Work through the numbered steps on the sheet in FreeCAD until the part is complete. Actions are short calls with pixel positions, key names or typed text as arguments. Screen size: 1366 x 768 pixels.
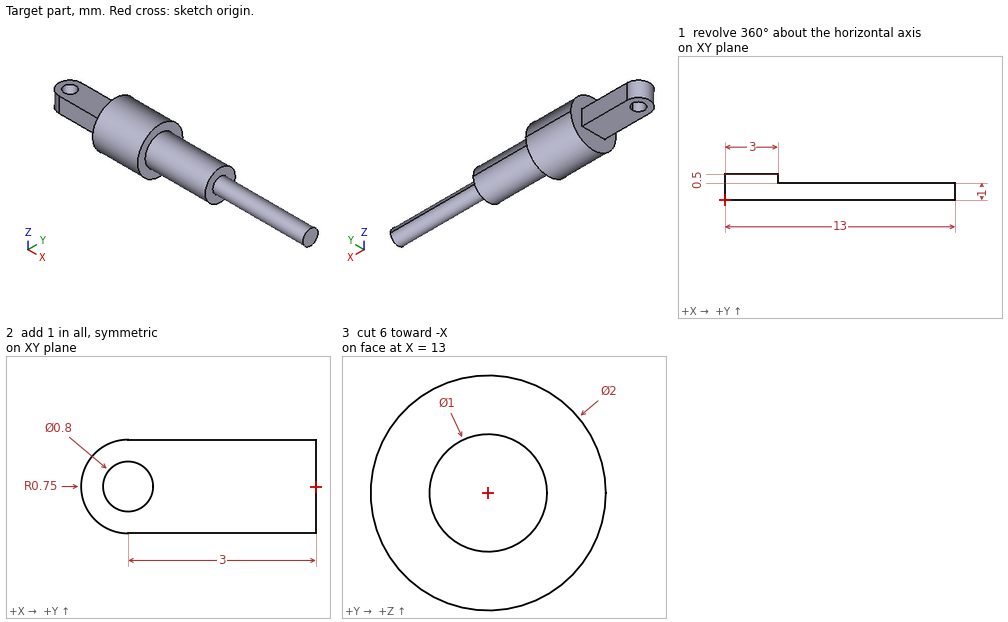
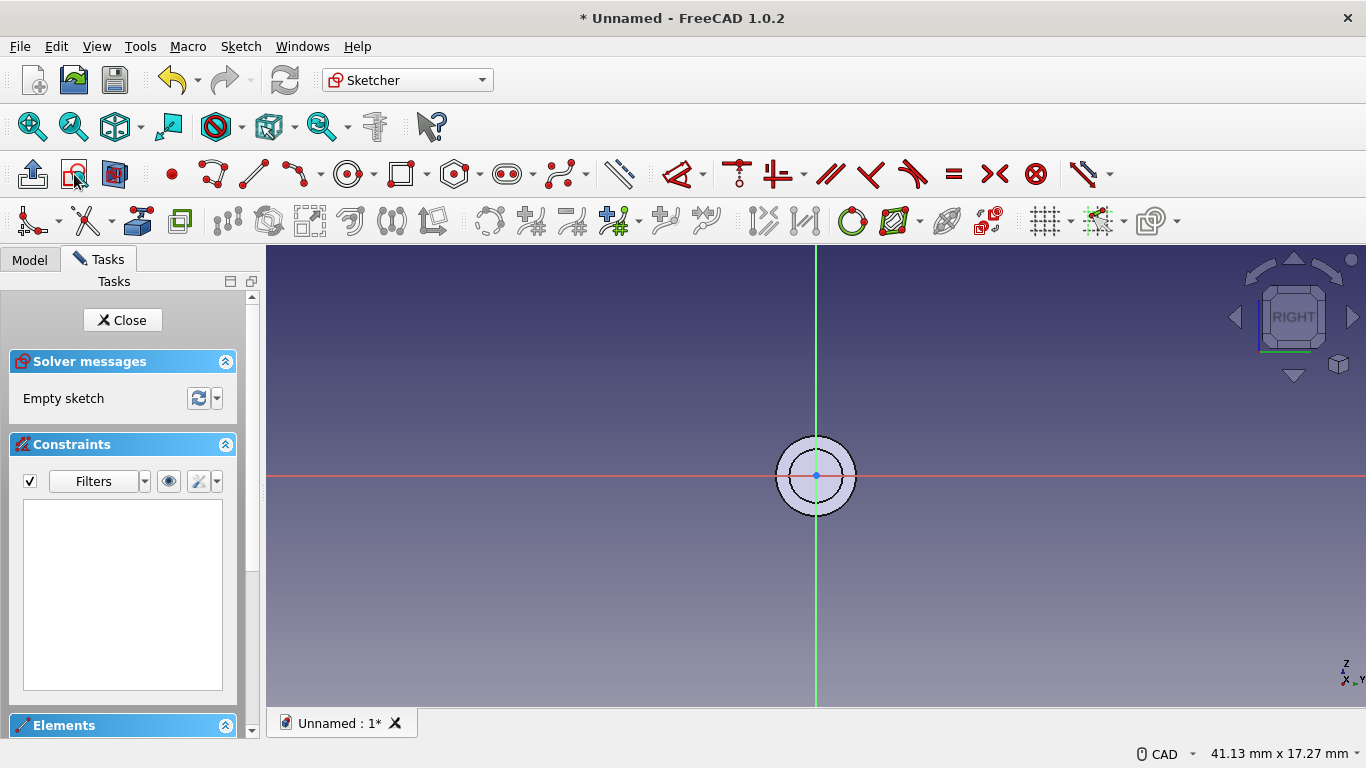
scroll(833, 476, up, 8)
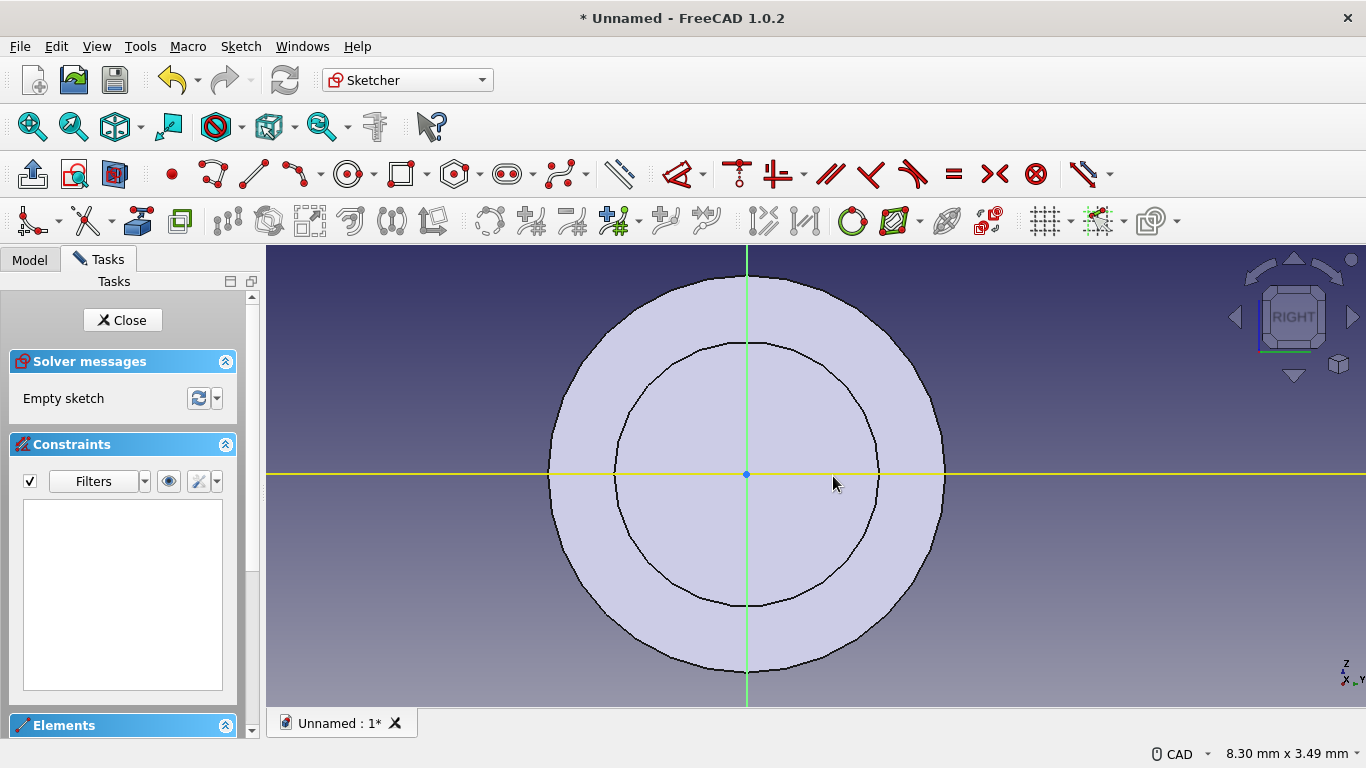
key(g)
key(c)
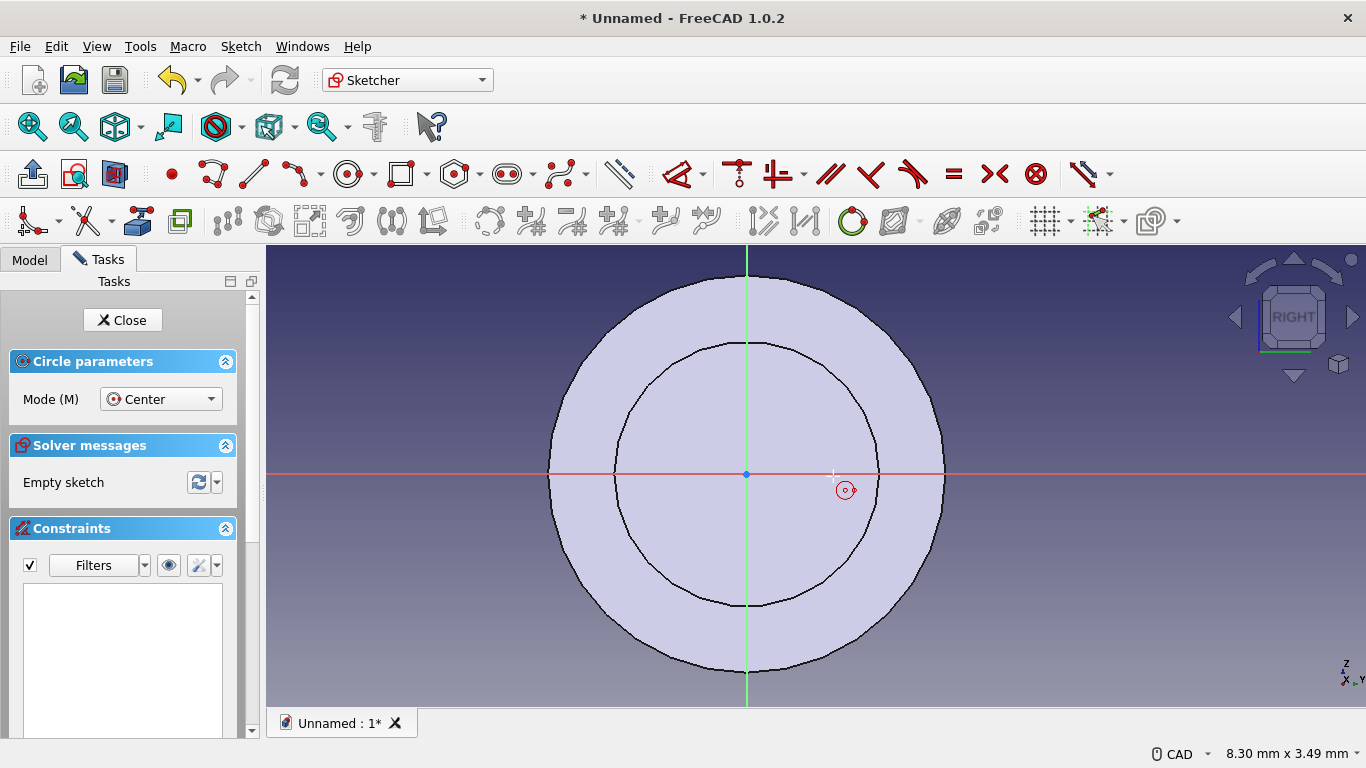
click(747, 474)
click(840, 380)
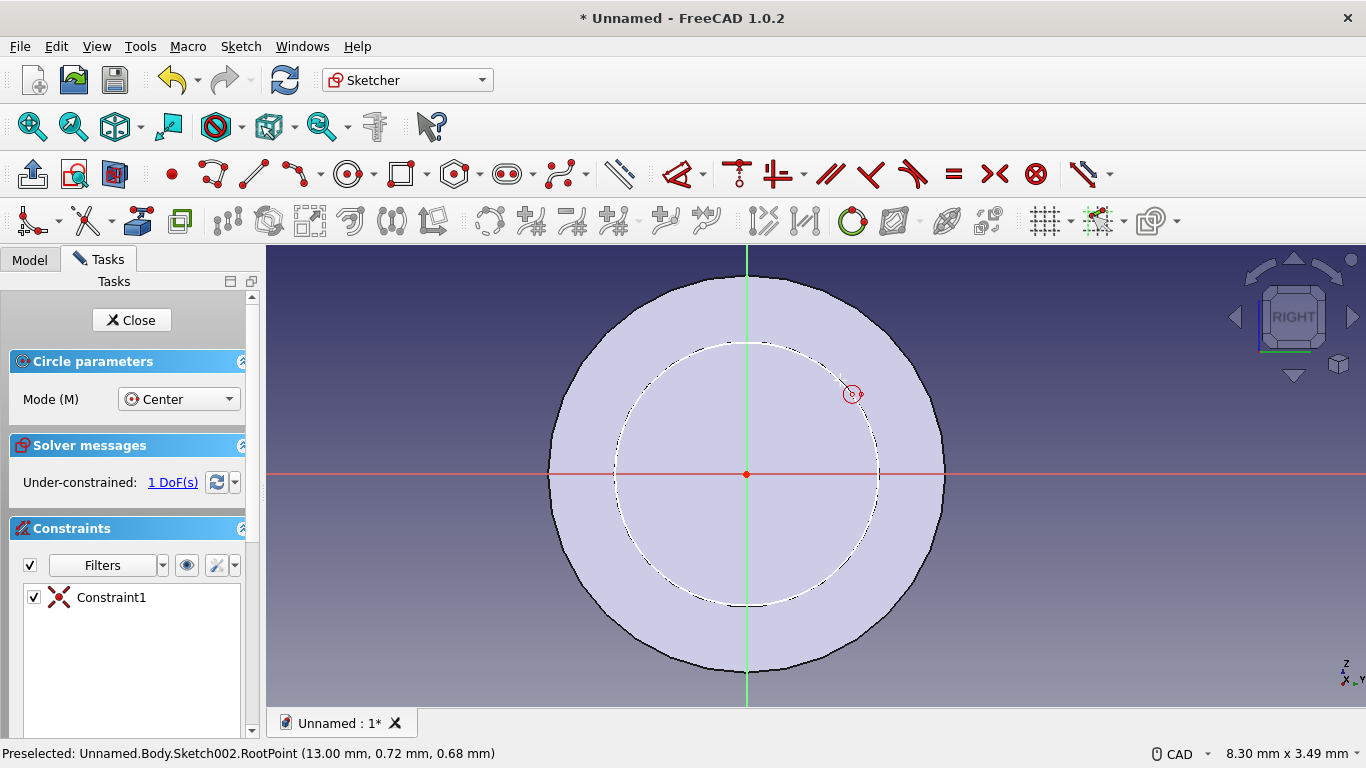
click(747, 474)
click(794, 427)
key(Escape)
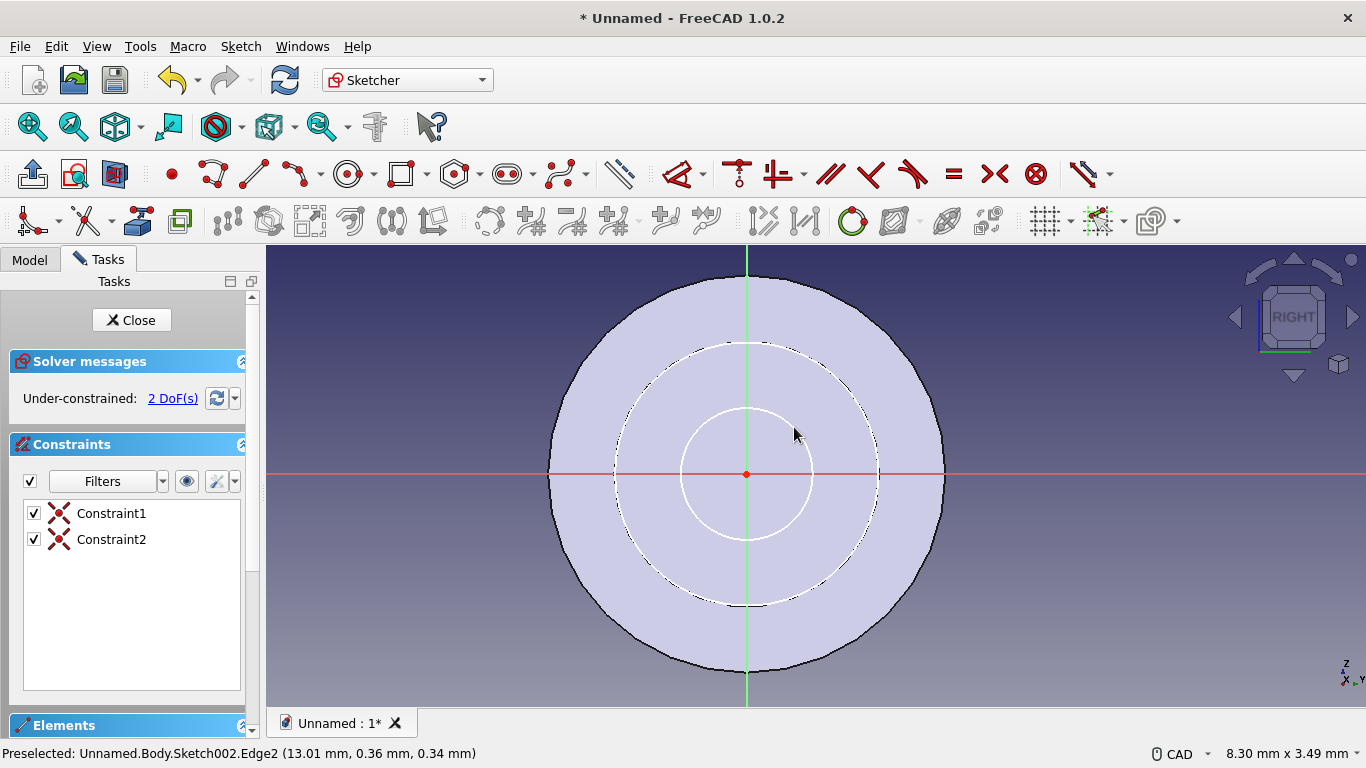
click(676, 174)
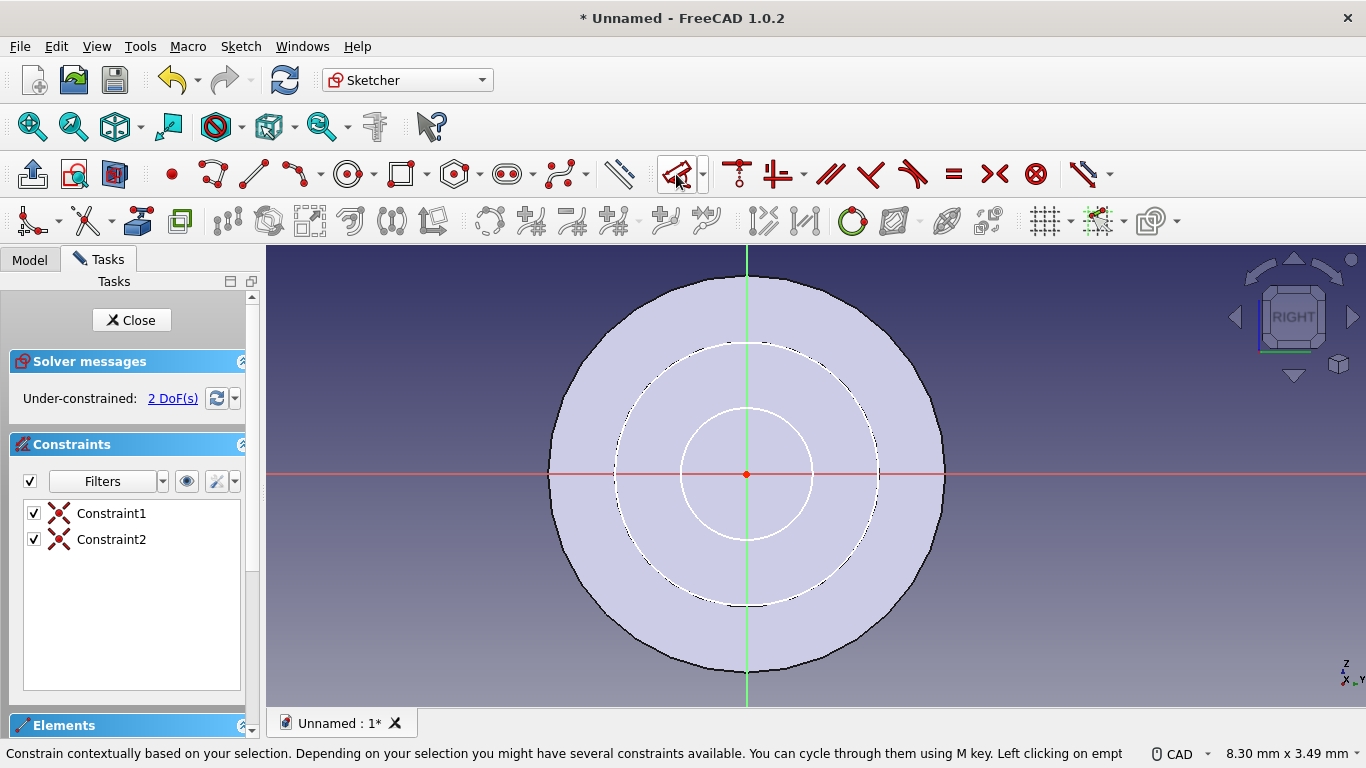
click(840, 381)
click(863, 358)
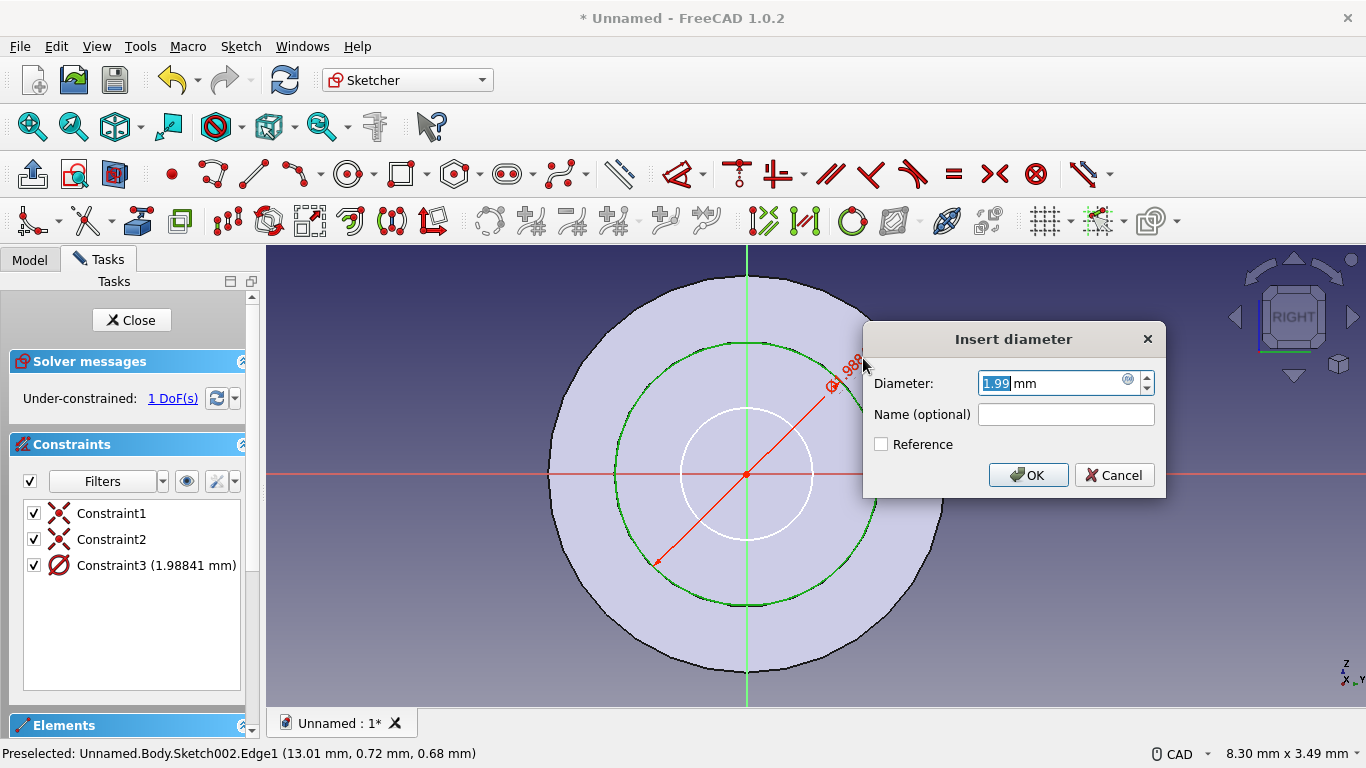
text(2)
key(Return)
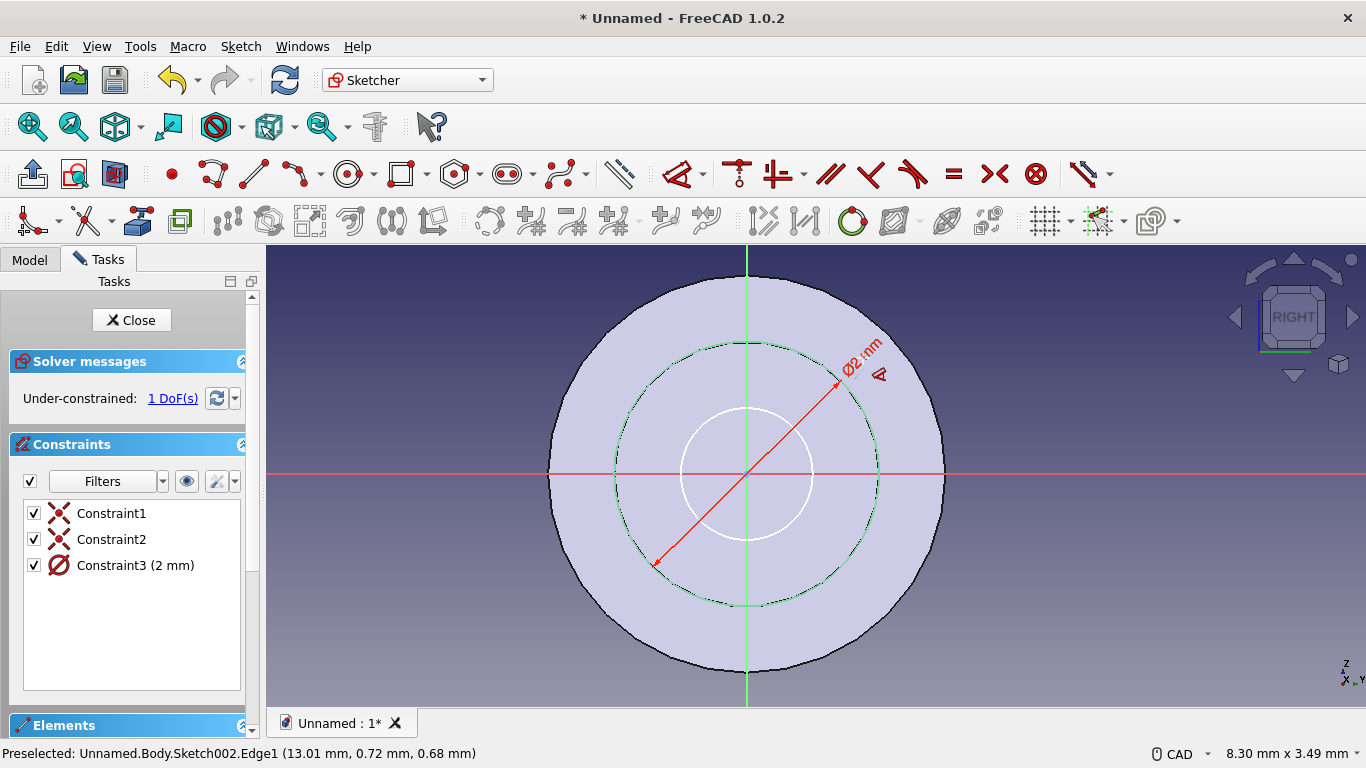
click(793, 427)
click(815, 404)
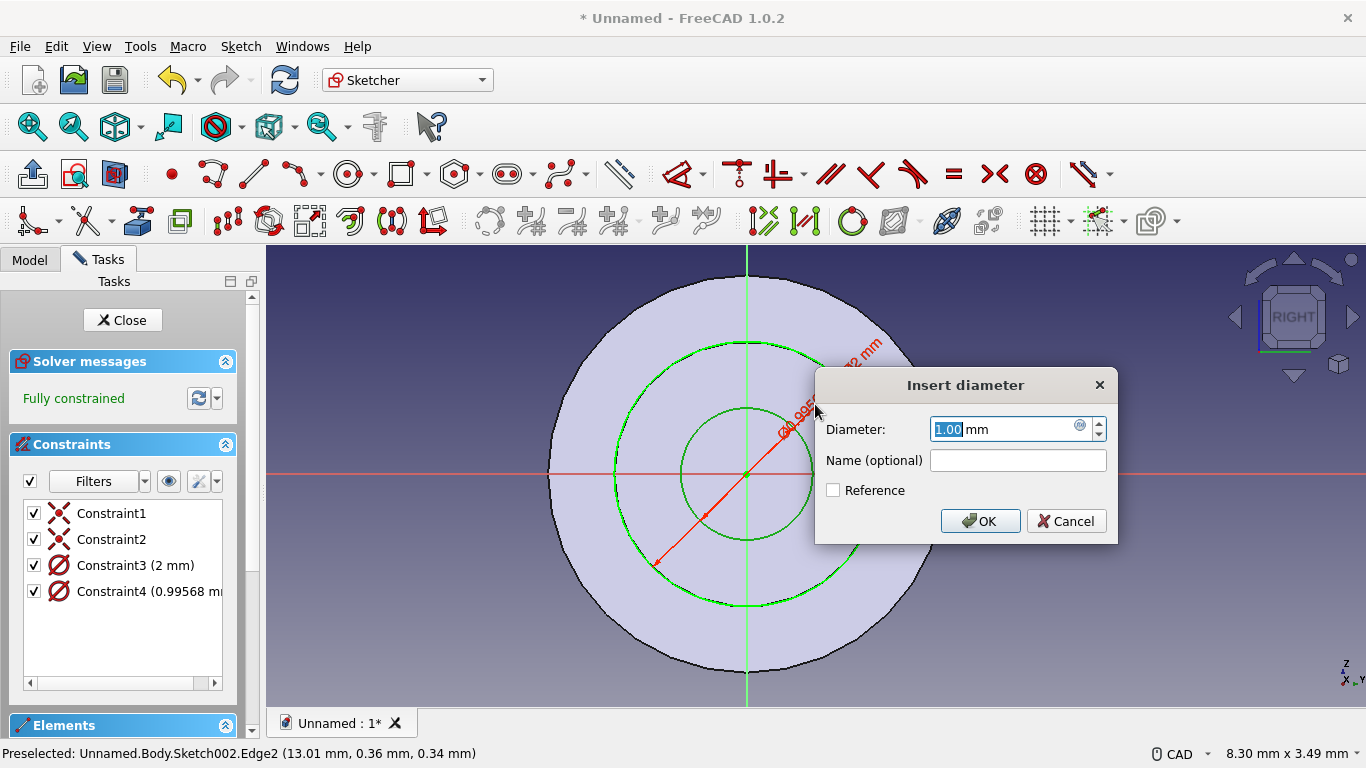
text(1)
key(Return)
key(Escape)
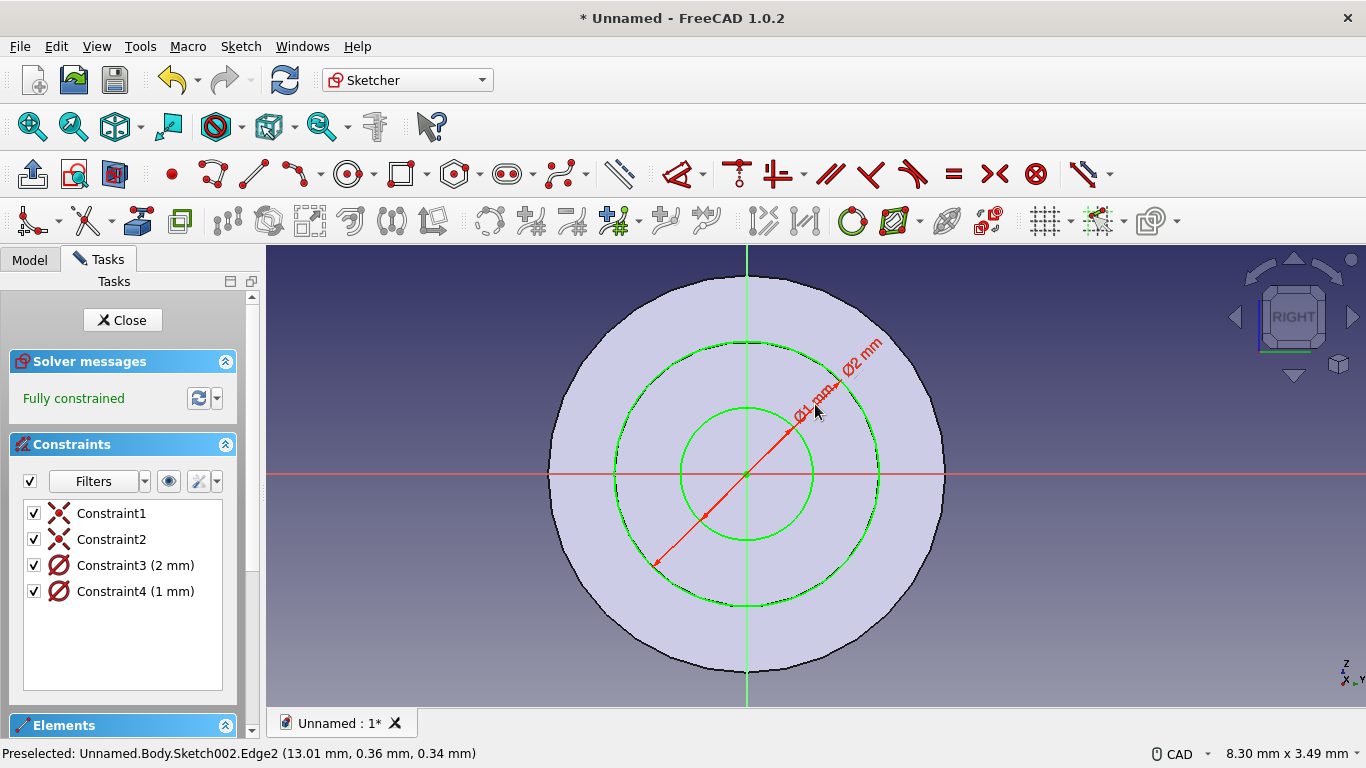
click(123, 320)